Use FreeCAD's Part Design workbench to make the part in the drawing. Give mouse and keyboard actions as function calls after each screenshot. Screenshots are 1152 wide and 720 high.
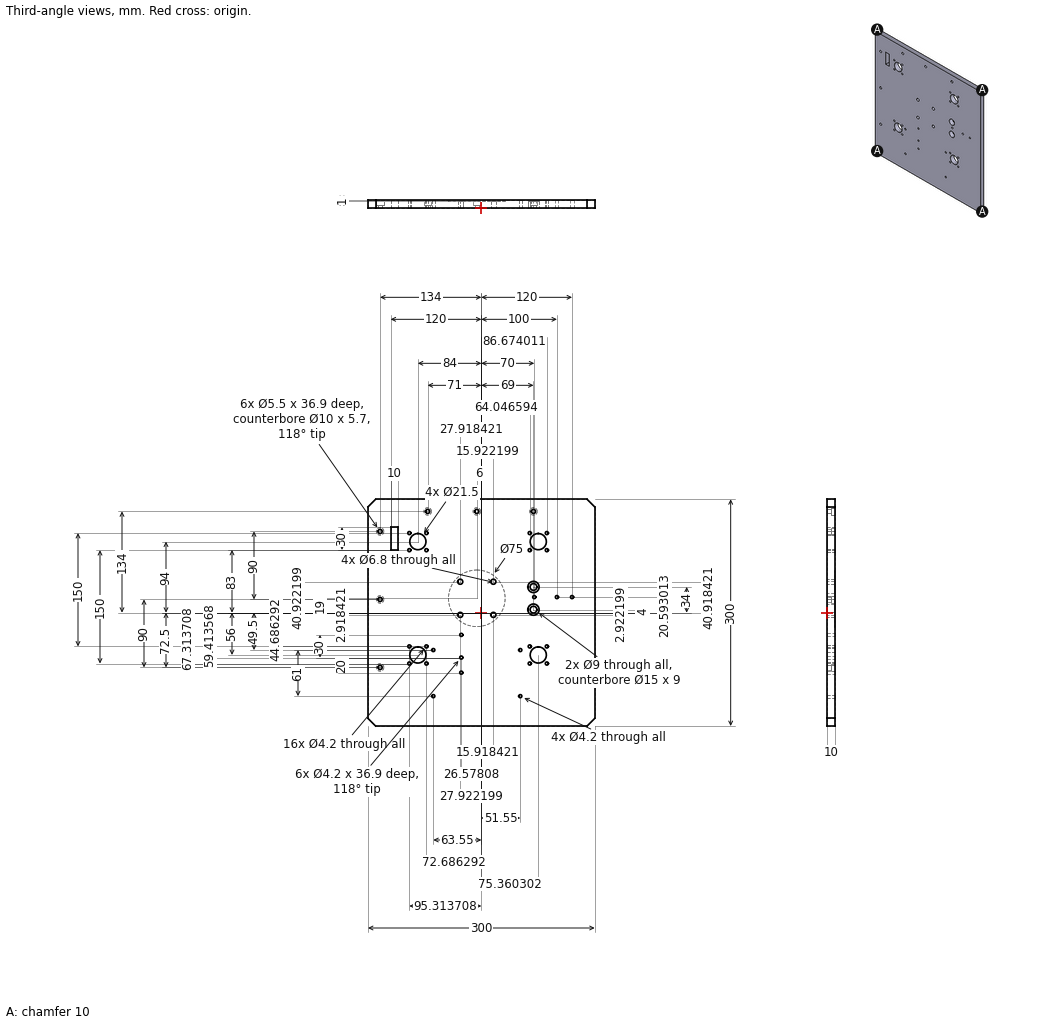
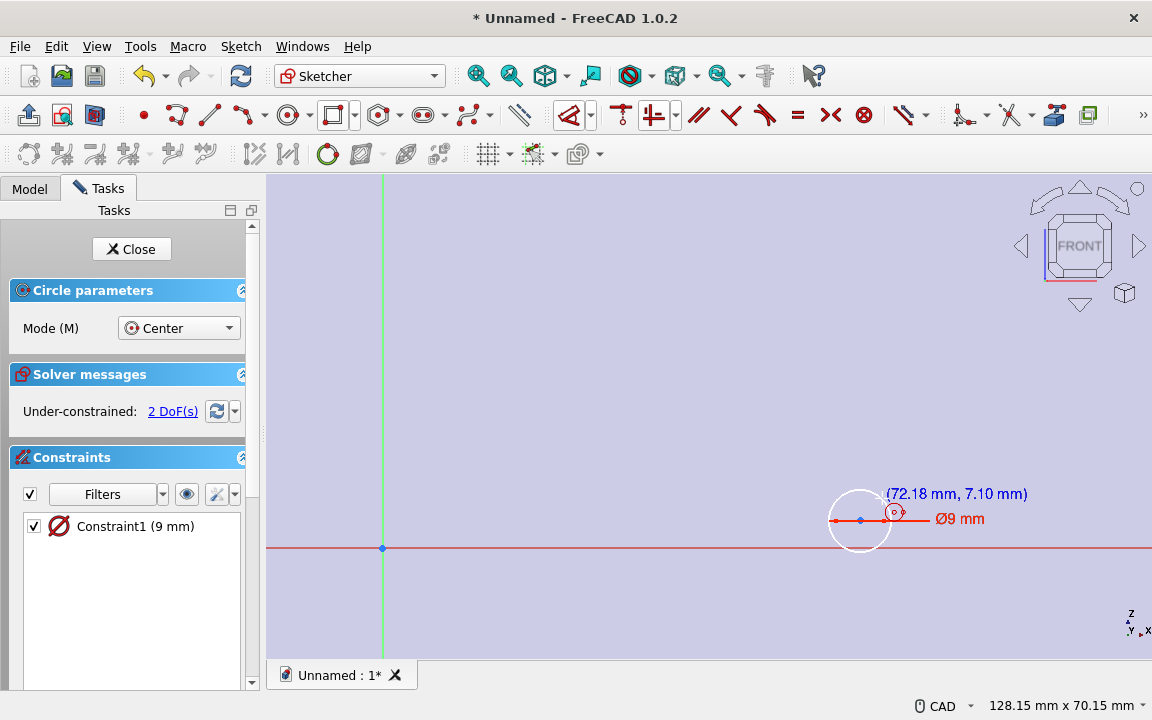
click(860, 313)
move(882, 291)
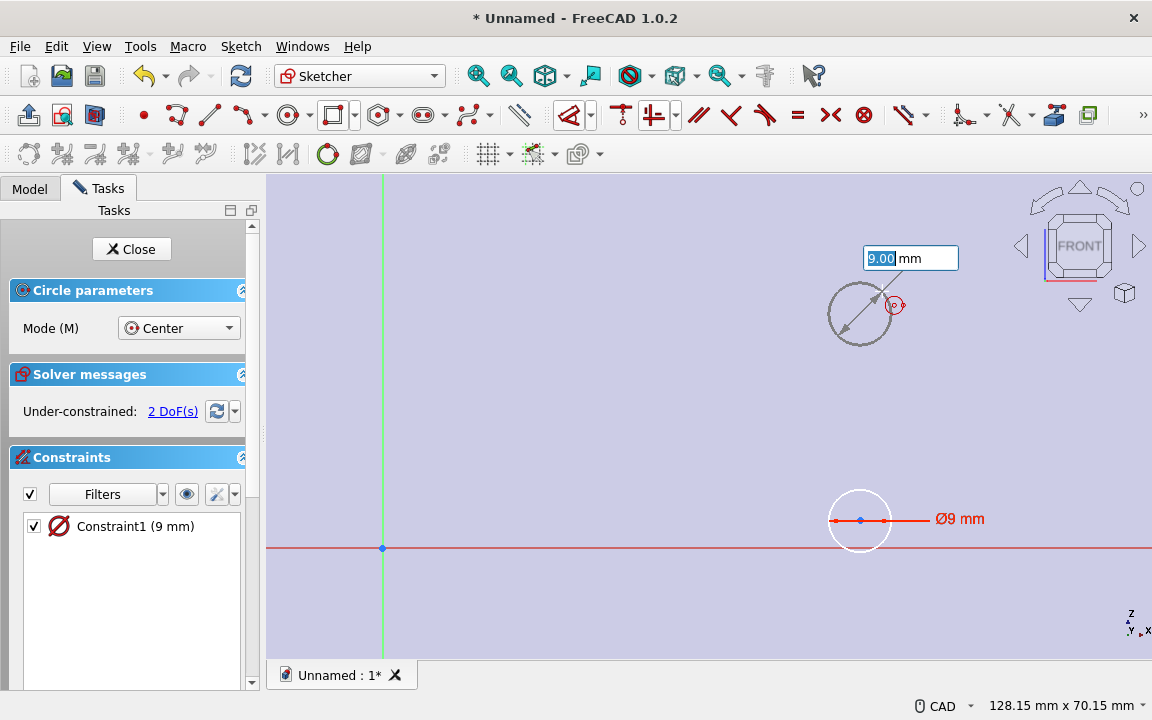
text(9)
key(Return)
key(Escape)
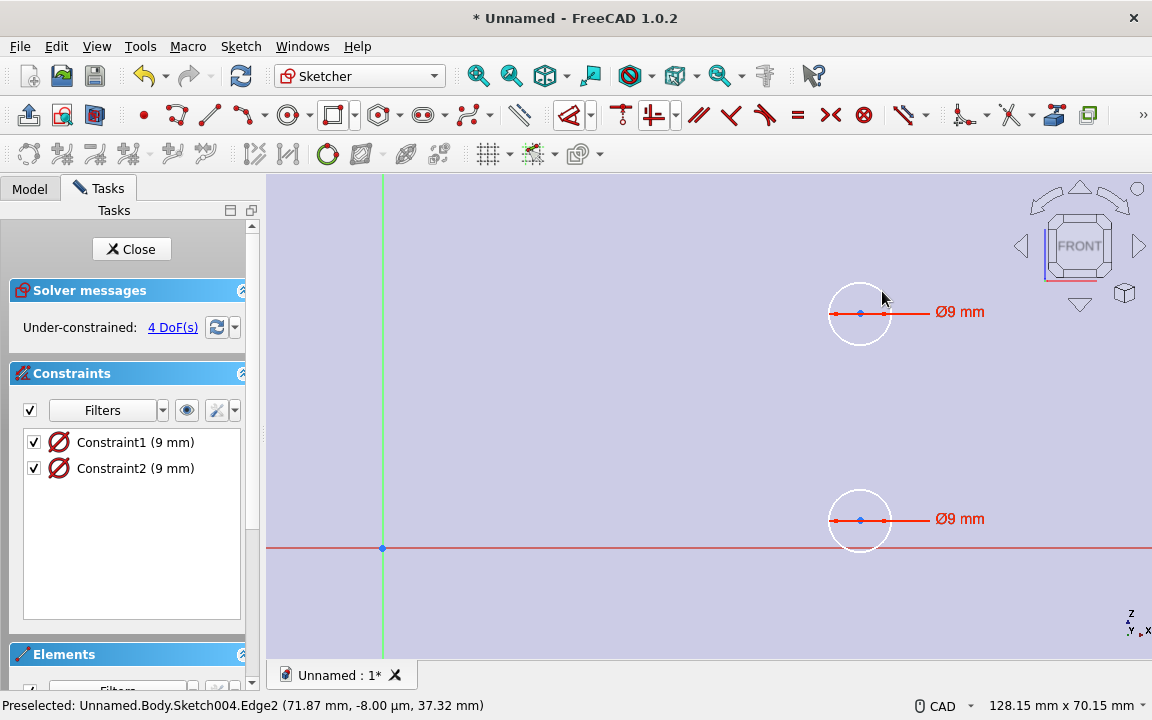
click(860, 521)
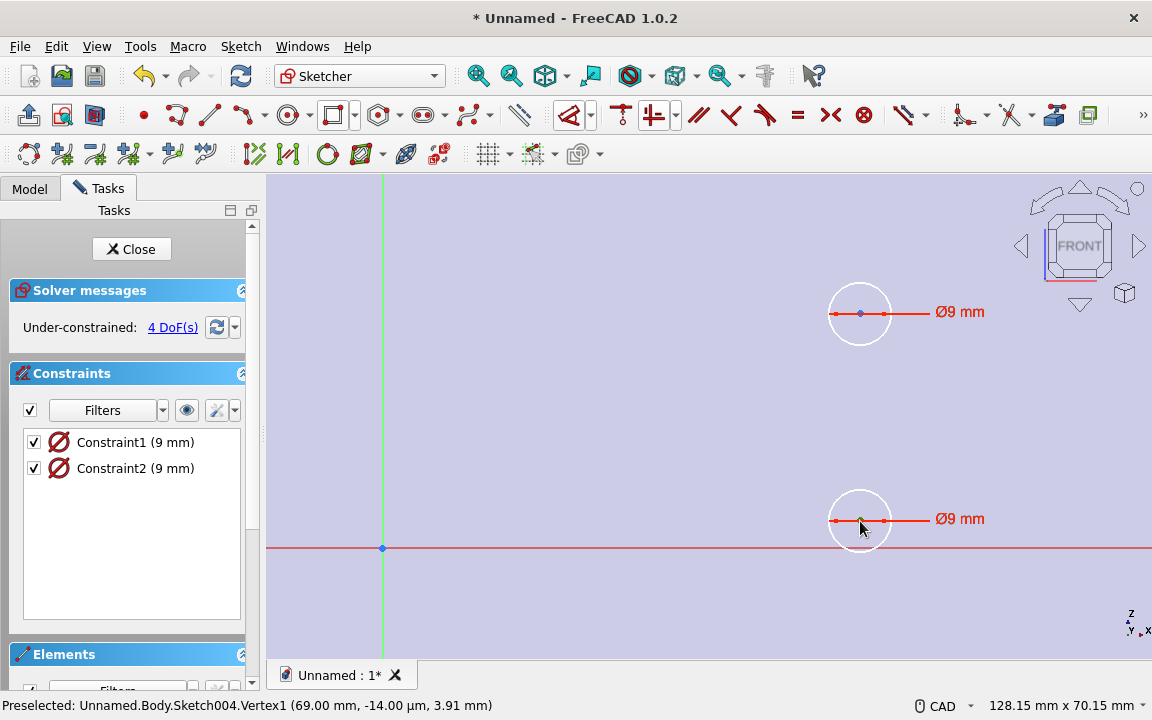
click(860, 314)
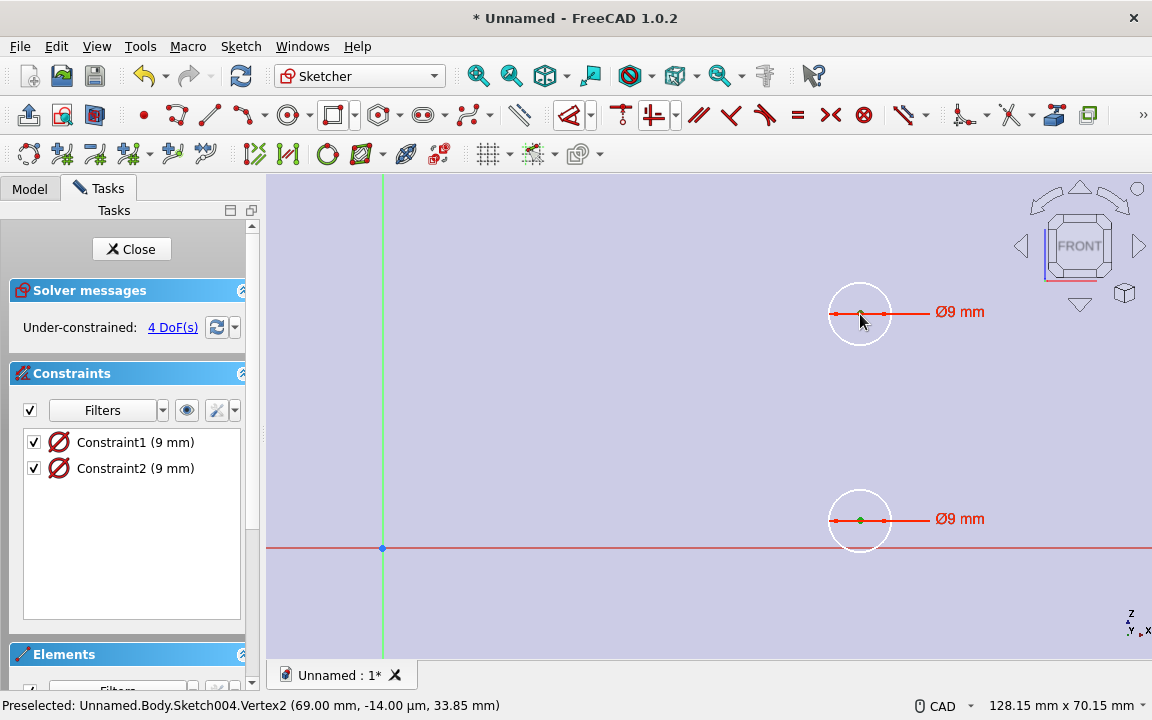
key(v)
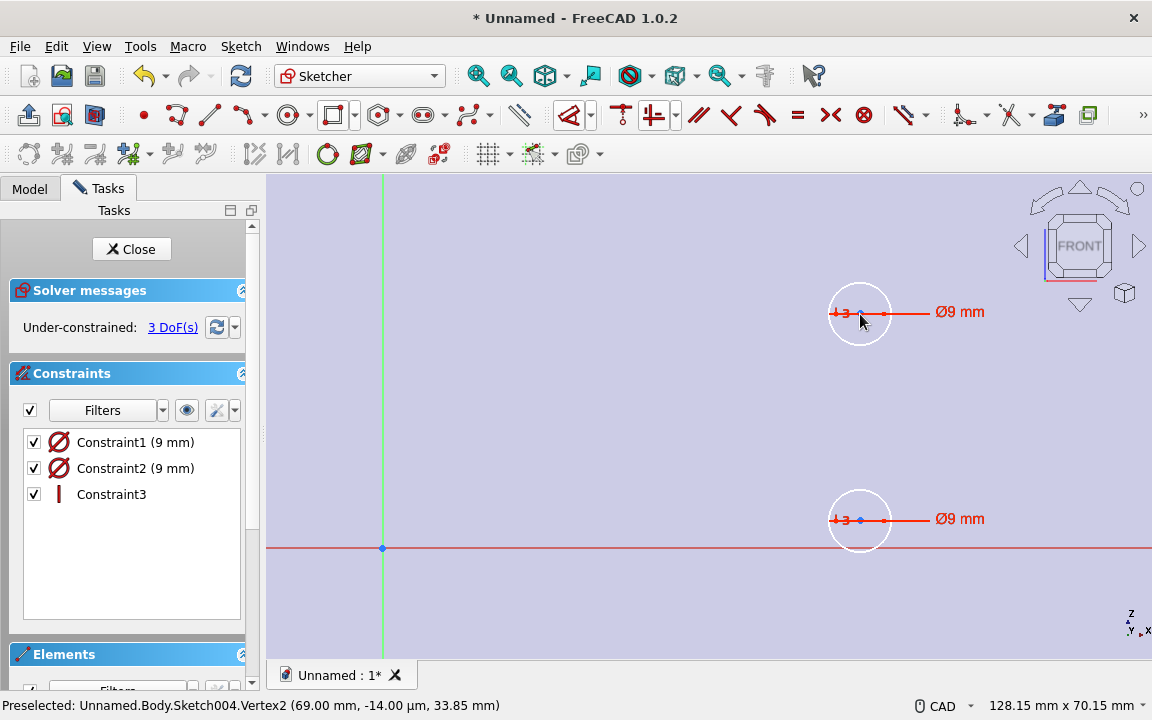
scroll(860, 521, up, 2)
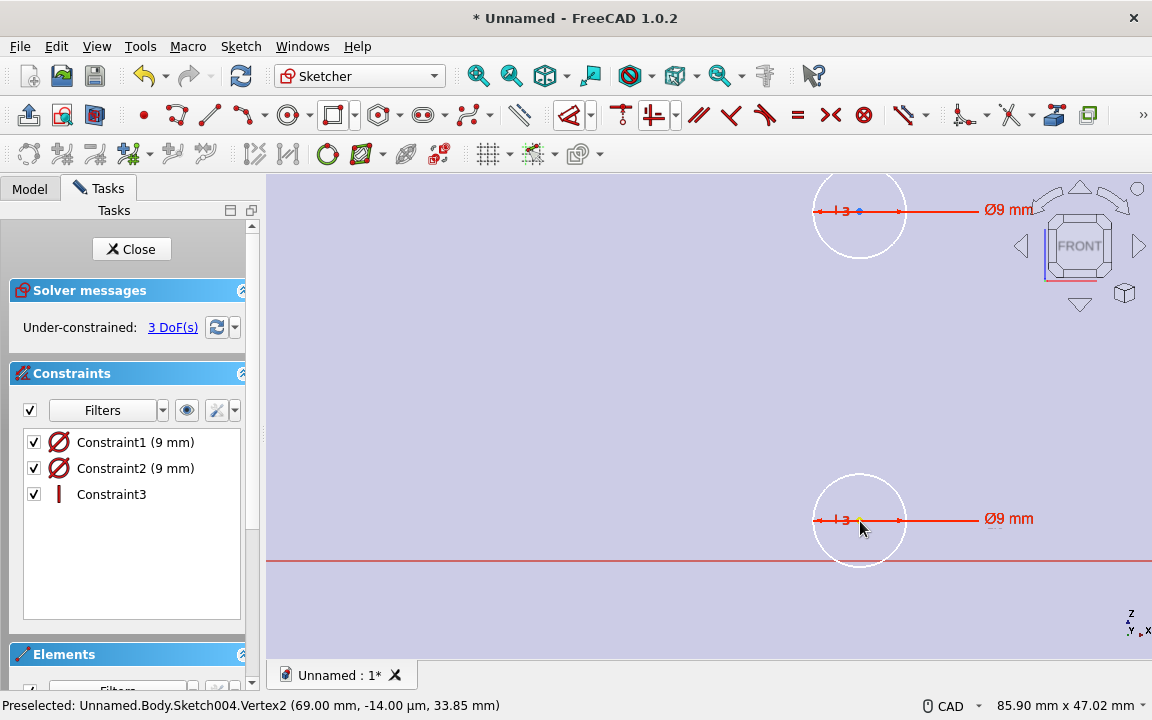
click(860, 521)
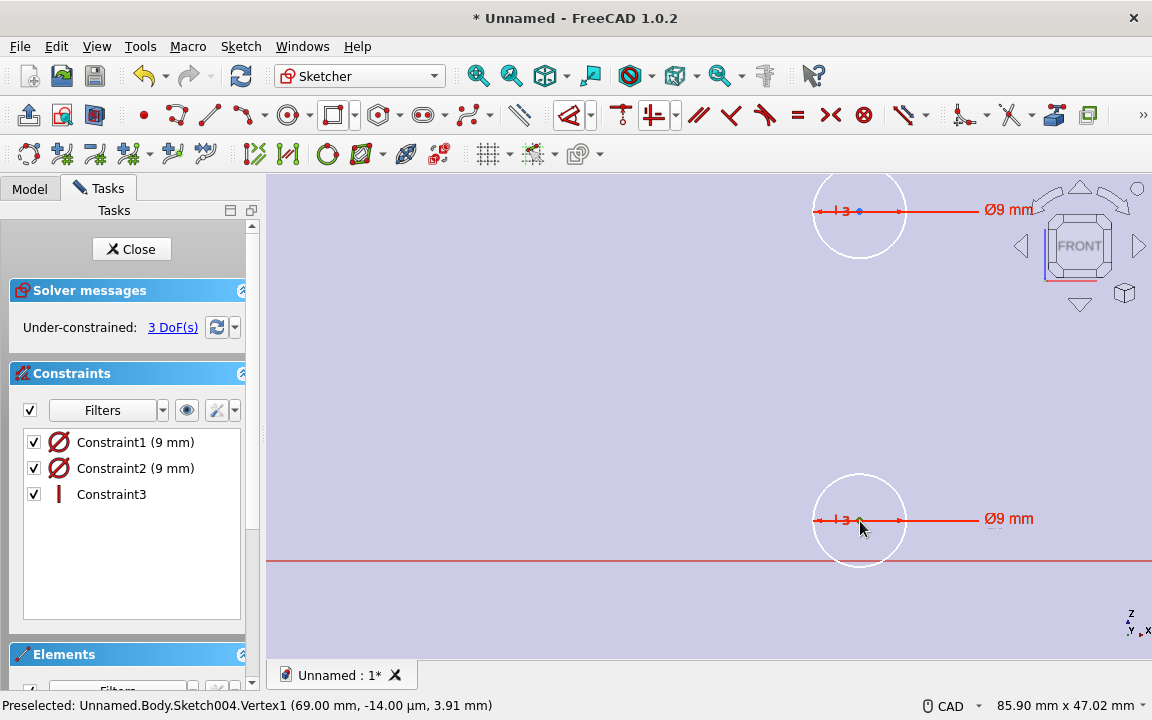
click(590, 116)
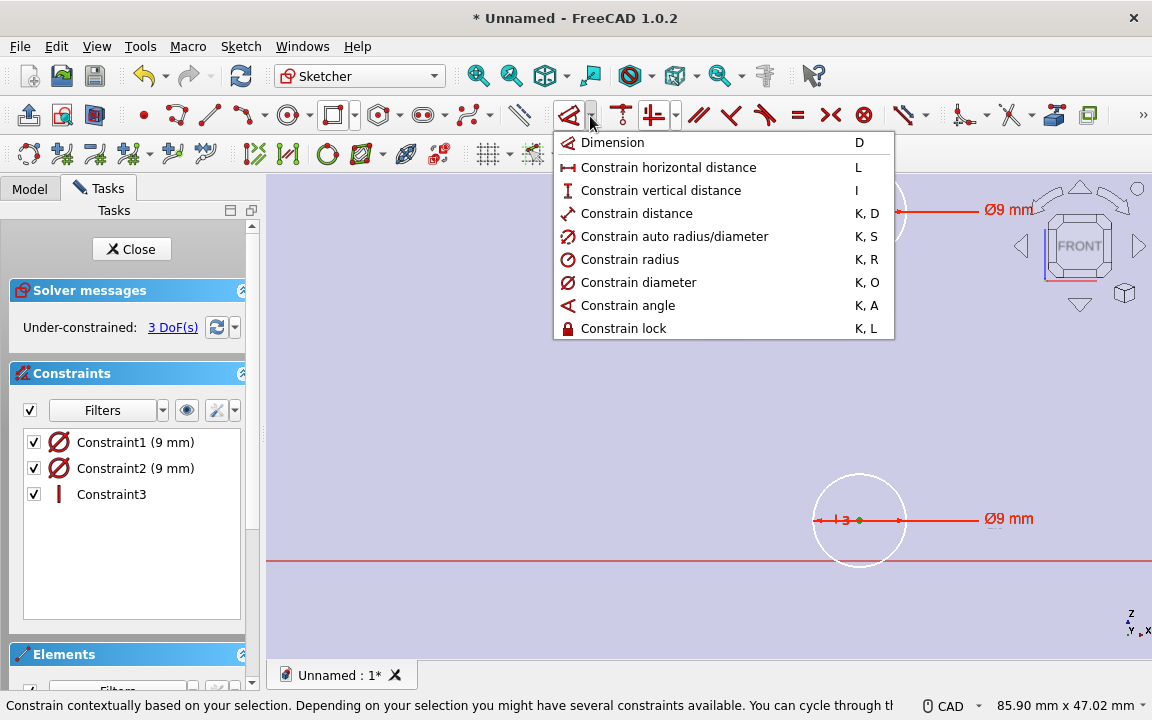
click(724, 190)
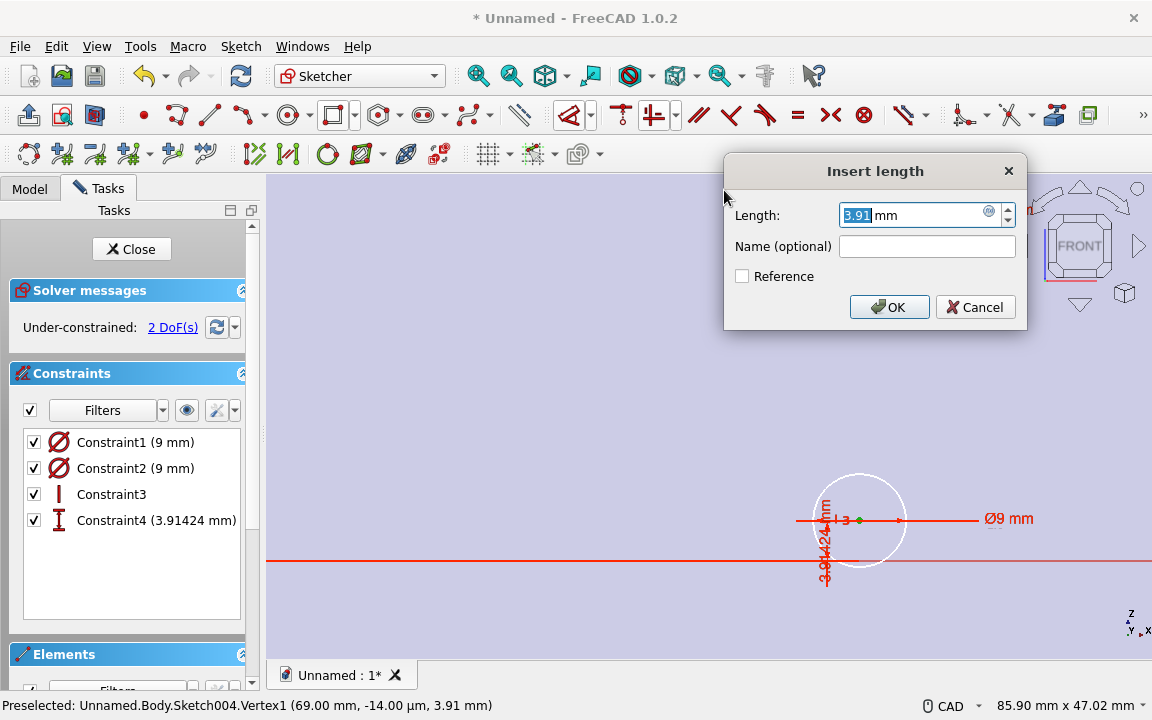
text(4)
key(Return)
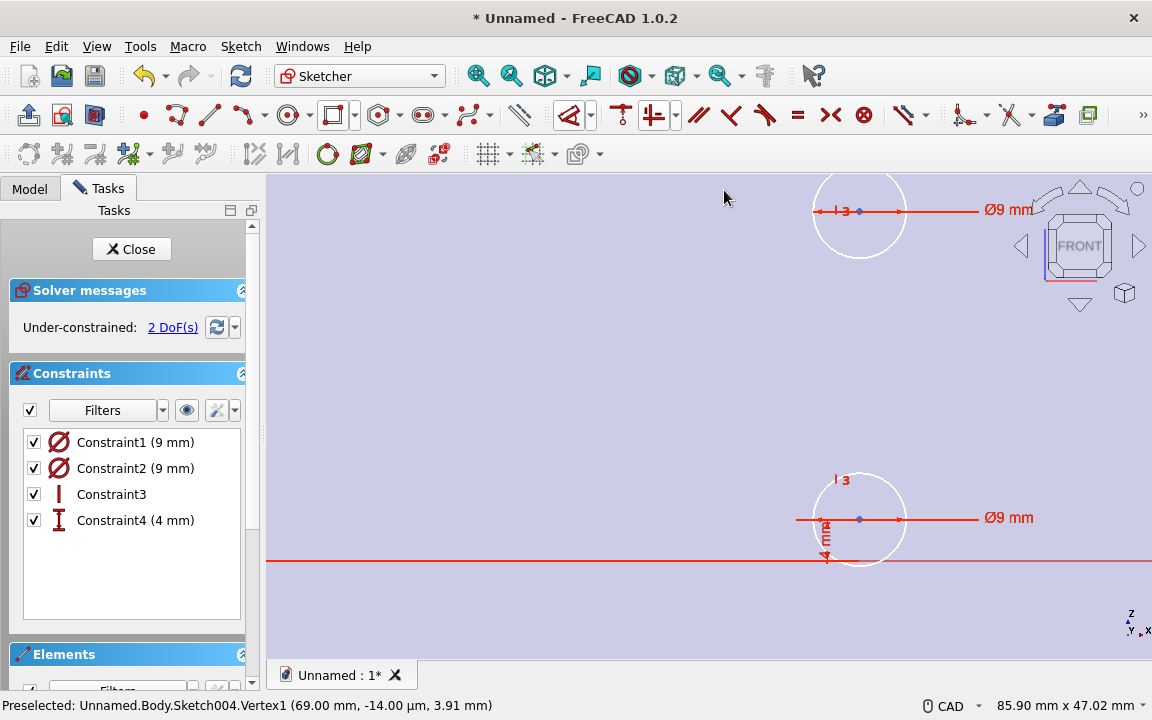
click(860, 520)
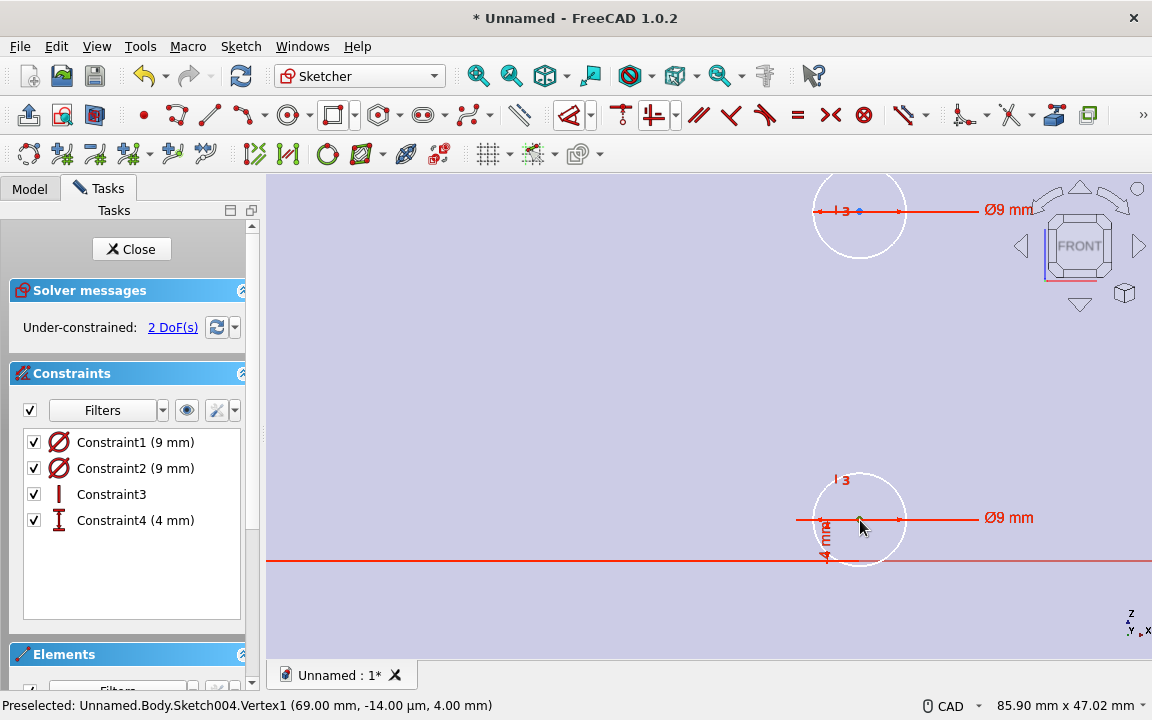
click(590, 116)